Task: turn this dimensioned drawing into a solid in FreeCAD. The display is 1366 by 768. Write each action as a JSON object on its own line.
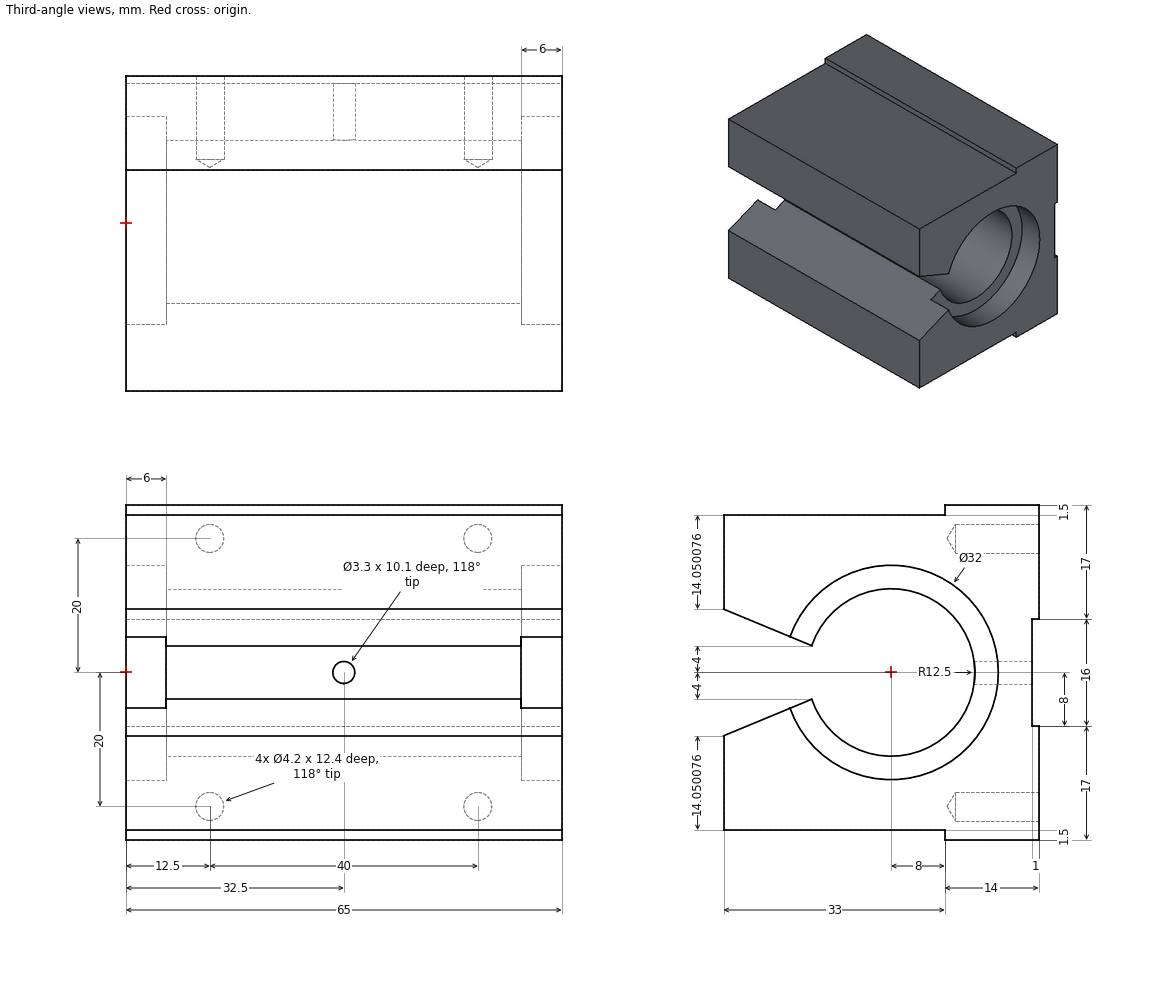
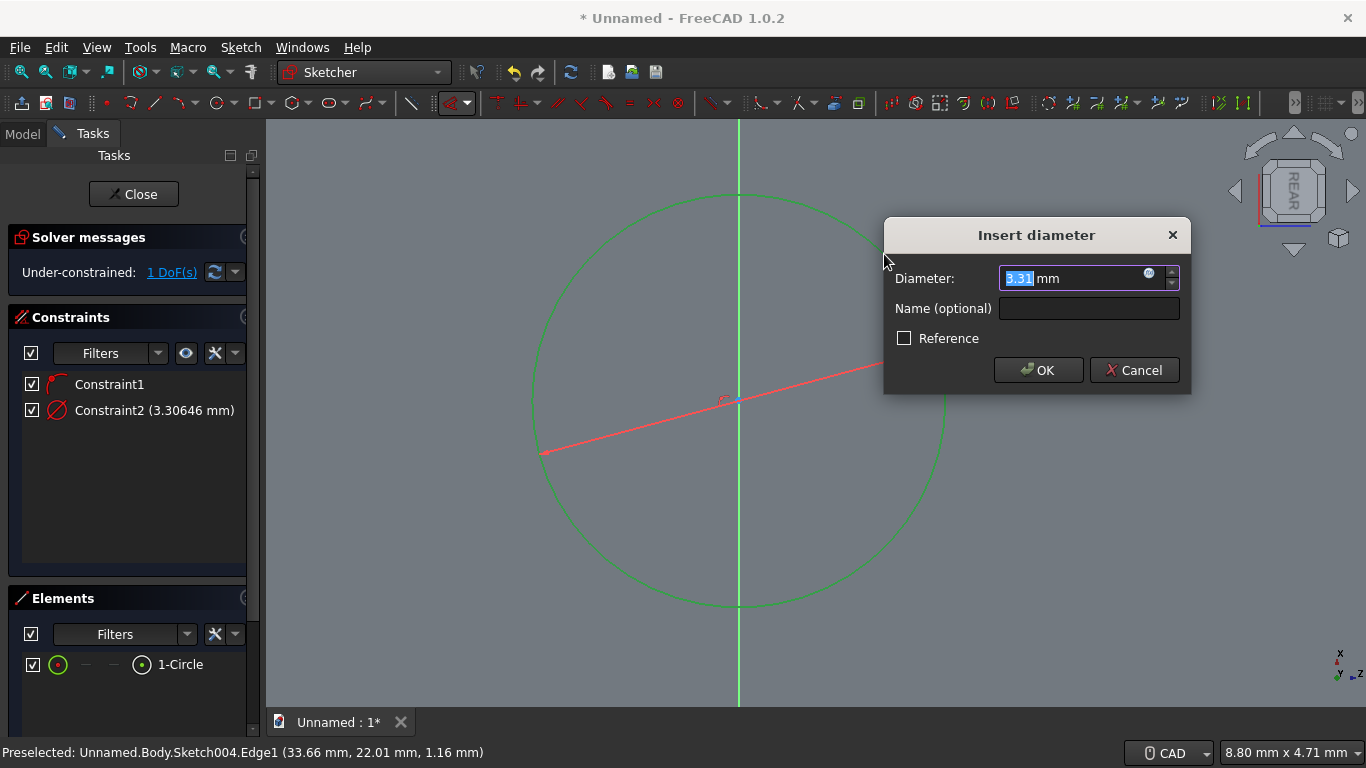
{"action": "type", "text": "3.3"}
{"action": "key", "text": "Return"}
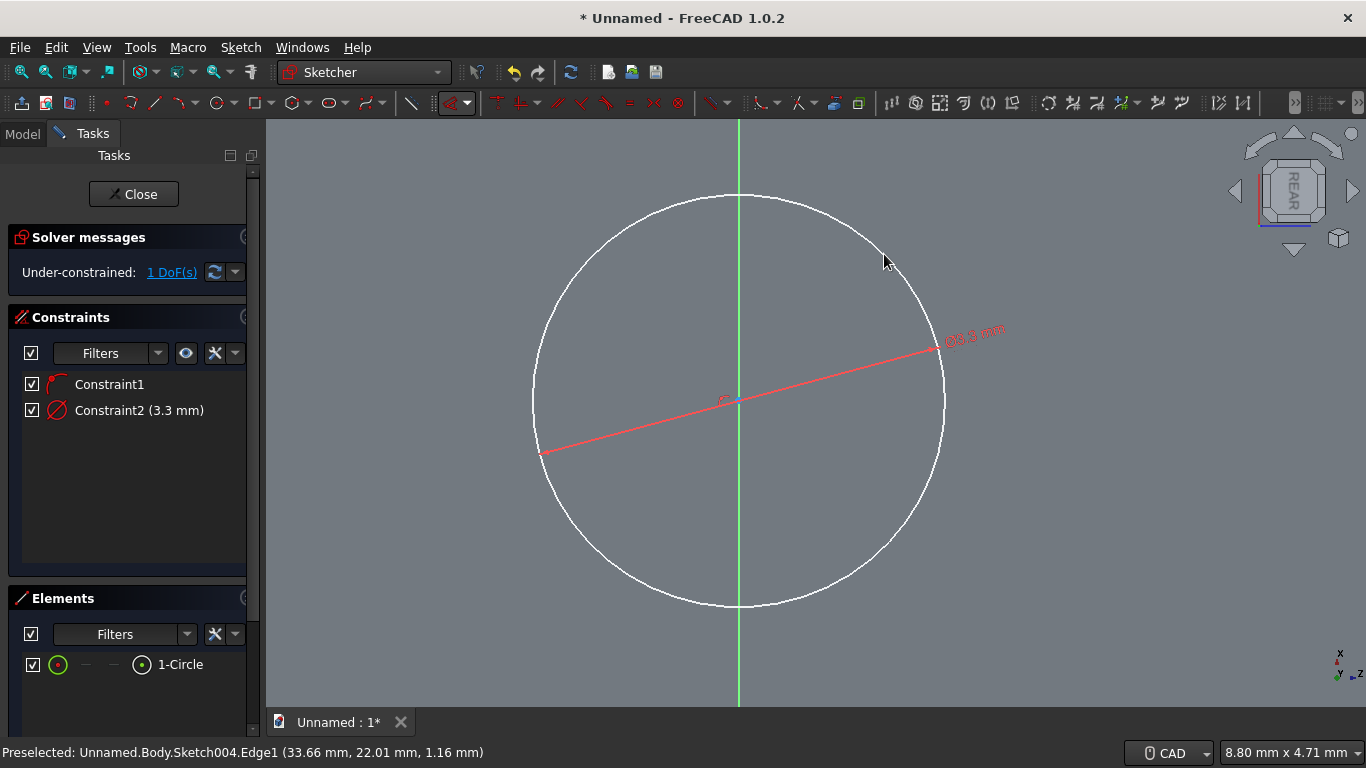
{"action": "left_click", "coordinate": [739, 401]}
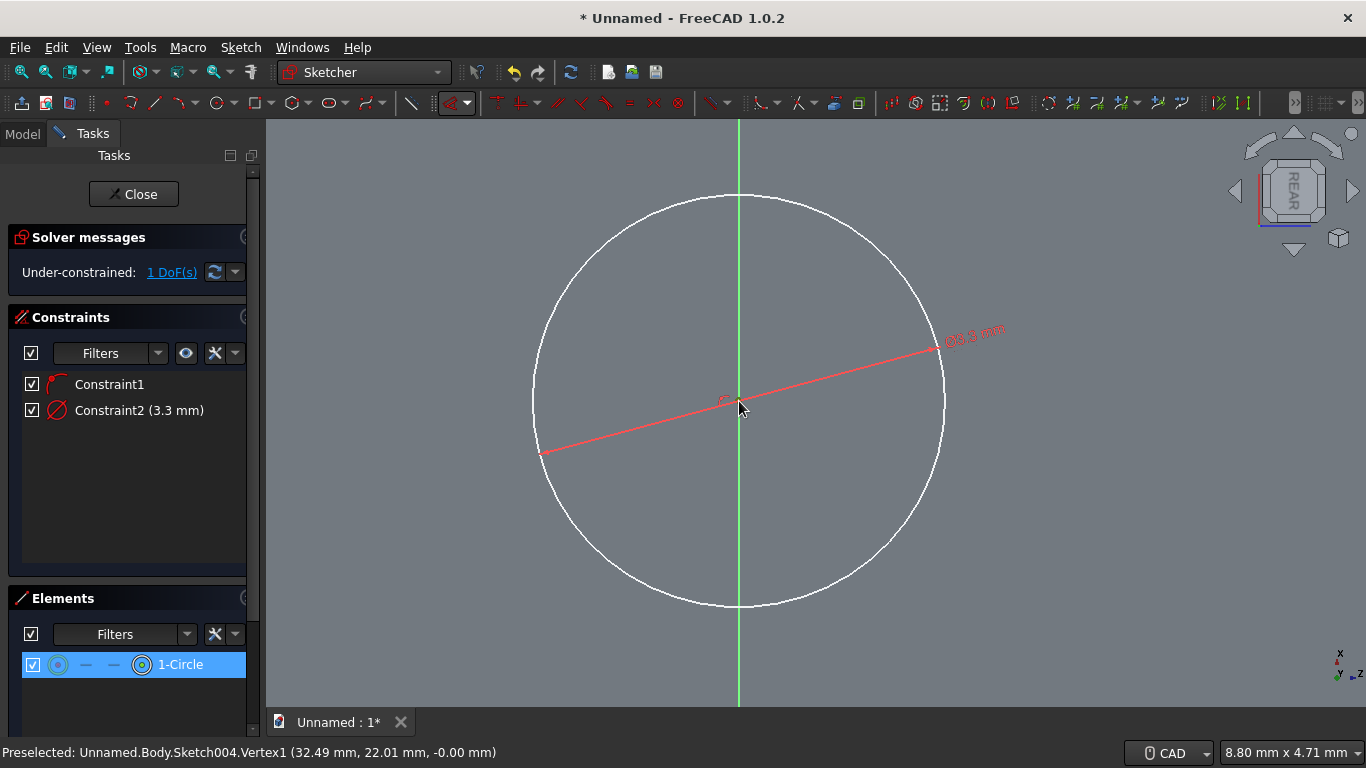
{"action": "key", "text": "i"}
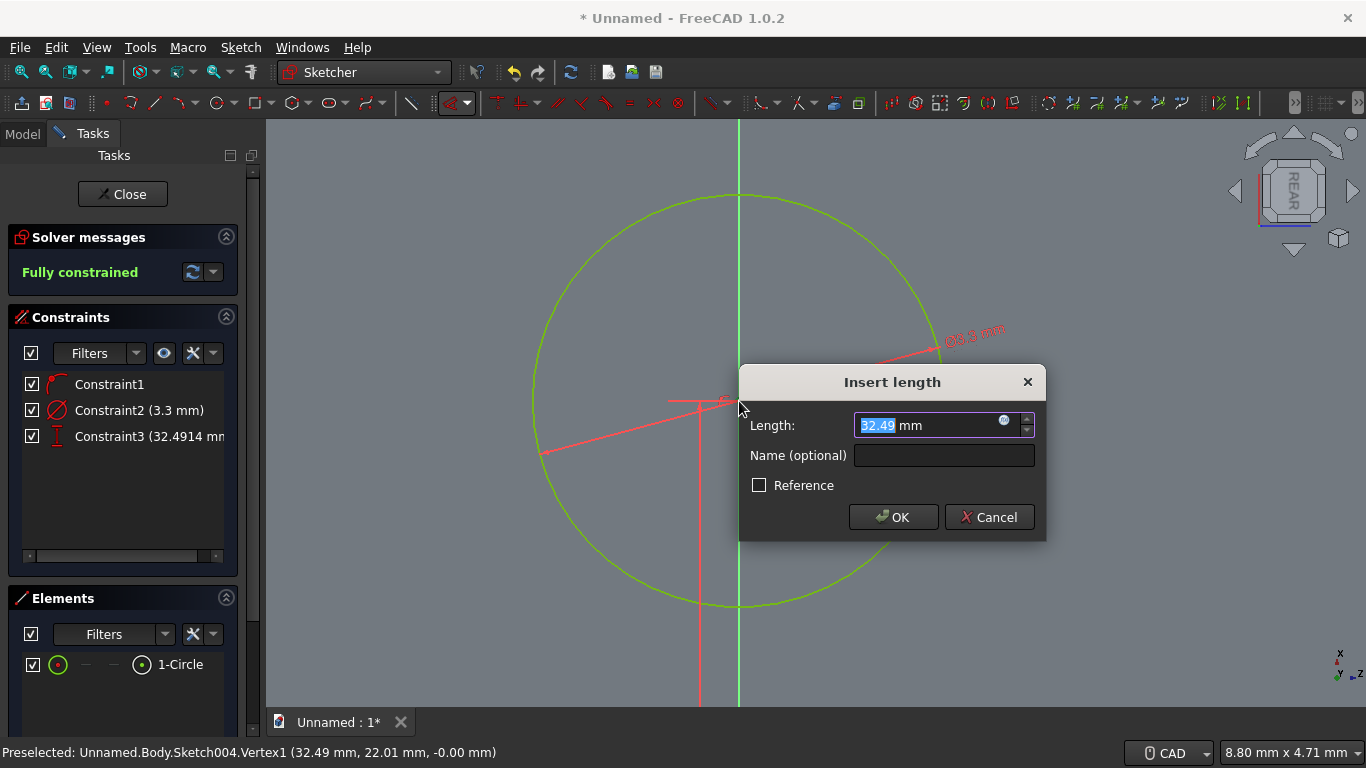
{"action": "type", "text": "32.5"}
{"action": "key", "text": "Return"}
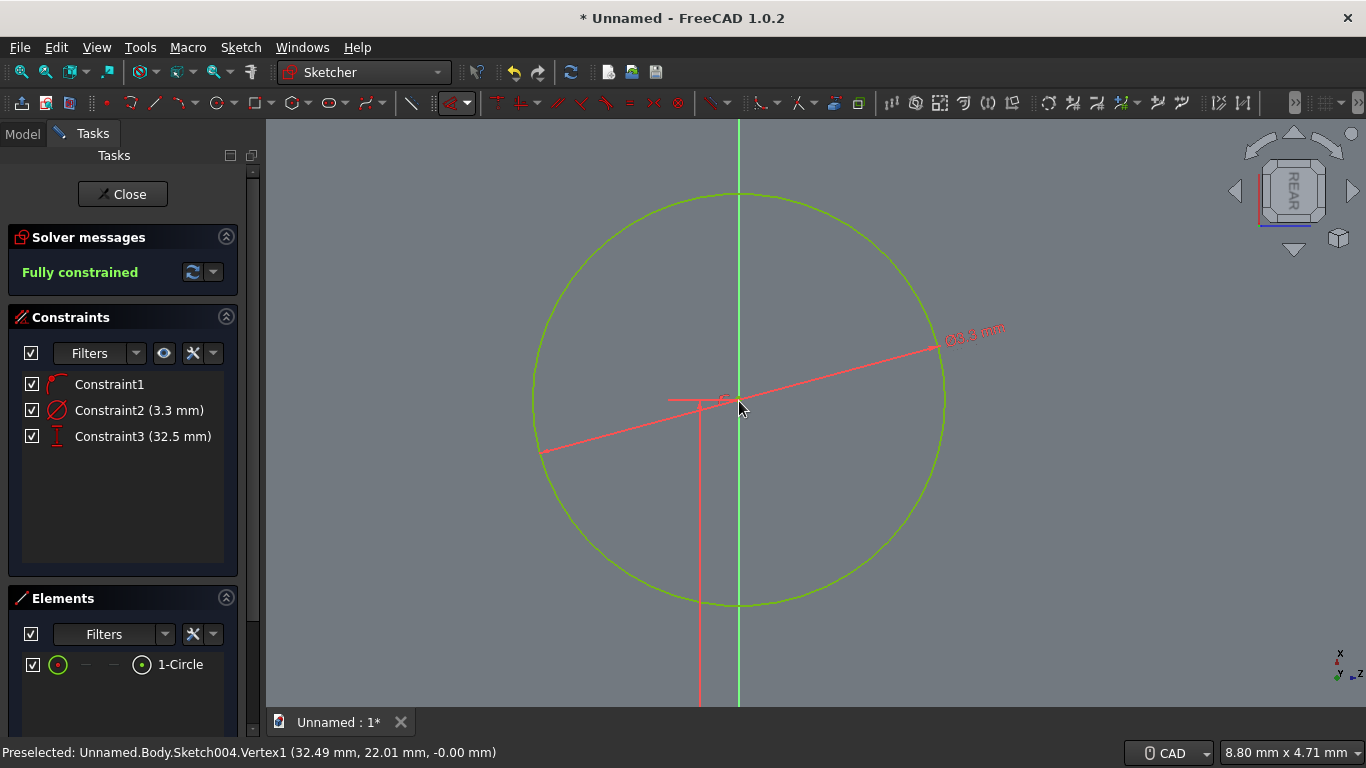
{"action": "left_click", "coordinate": [123, 194]}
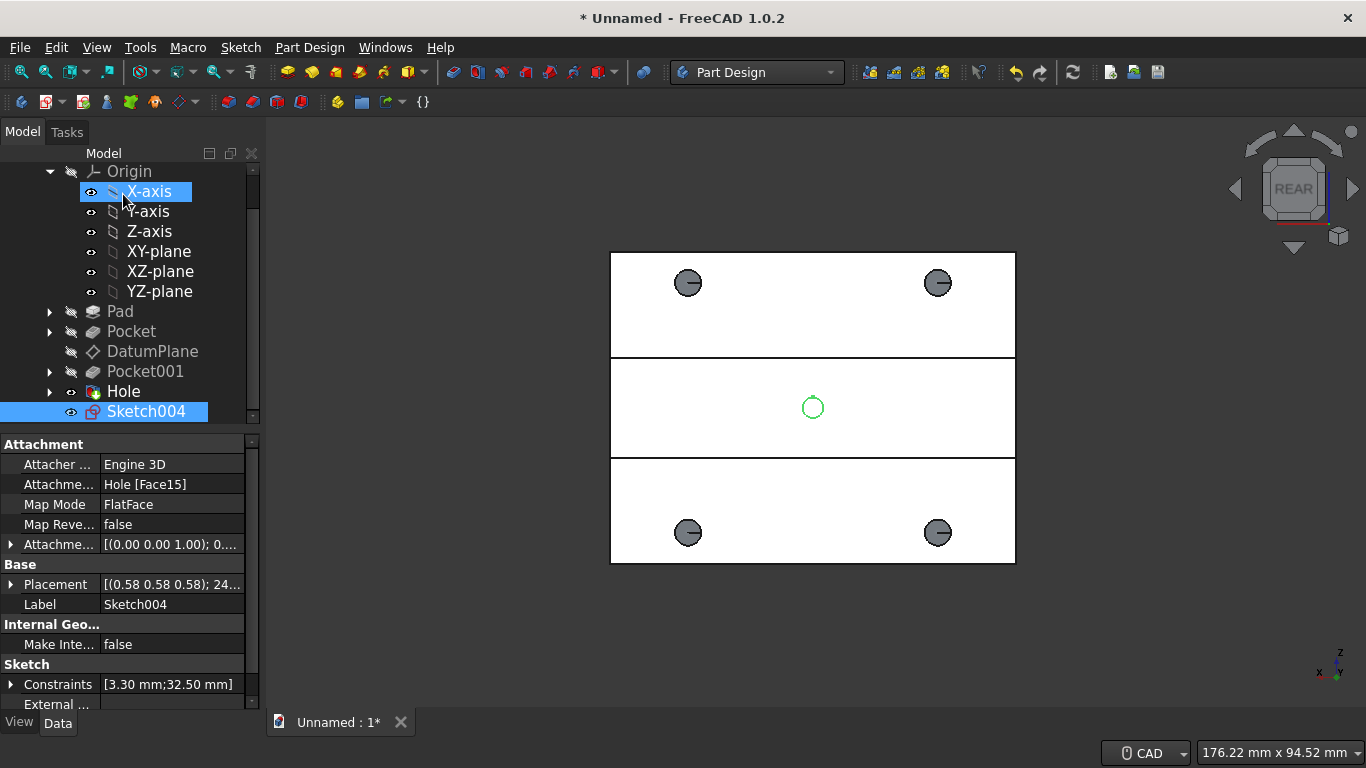
{"action": "left_click", "coordinate": [478, 72]}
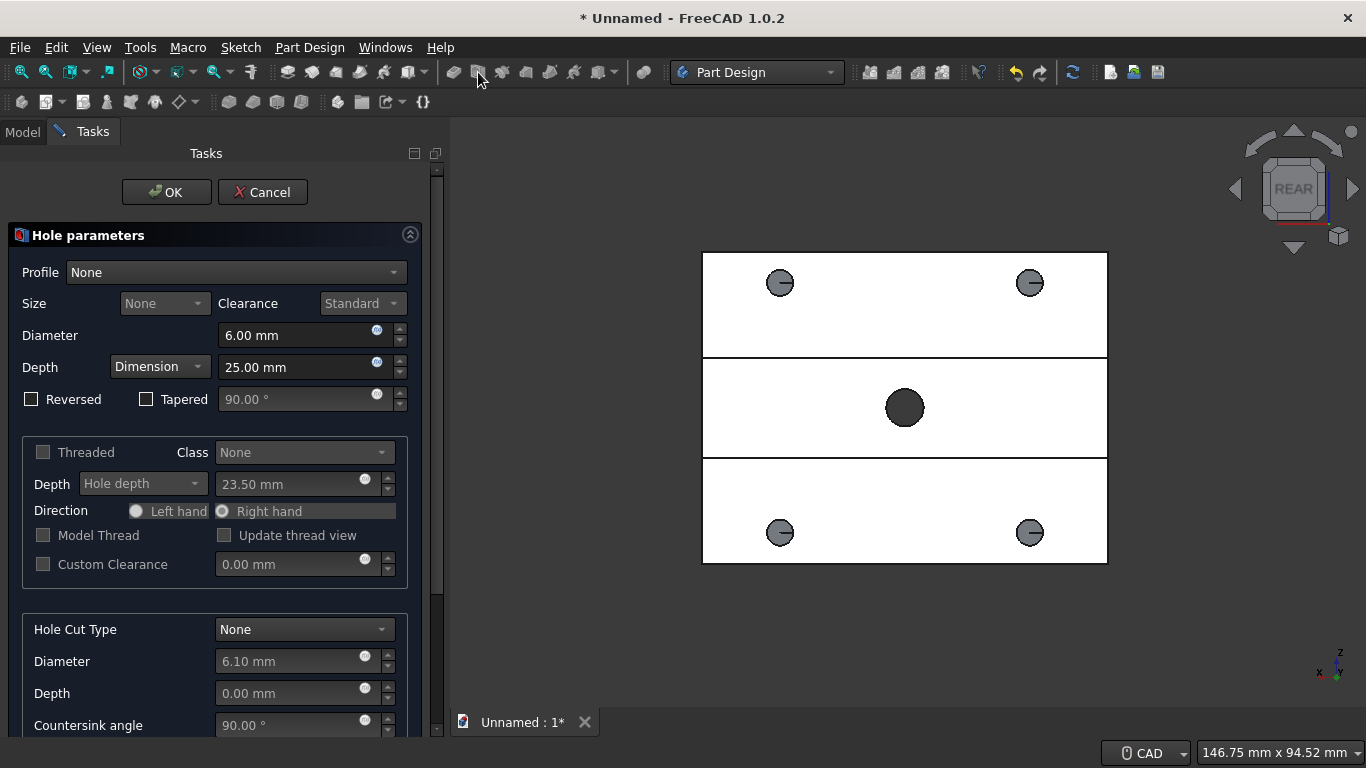
{"action": "triple_click", "coordinate": [305, 335]}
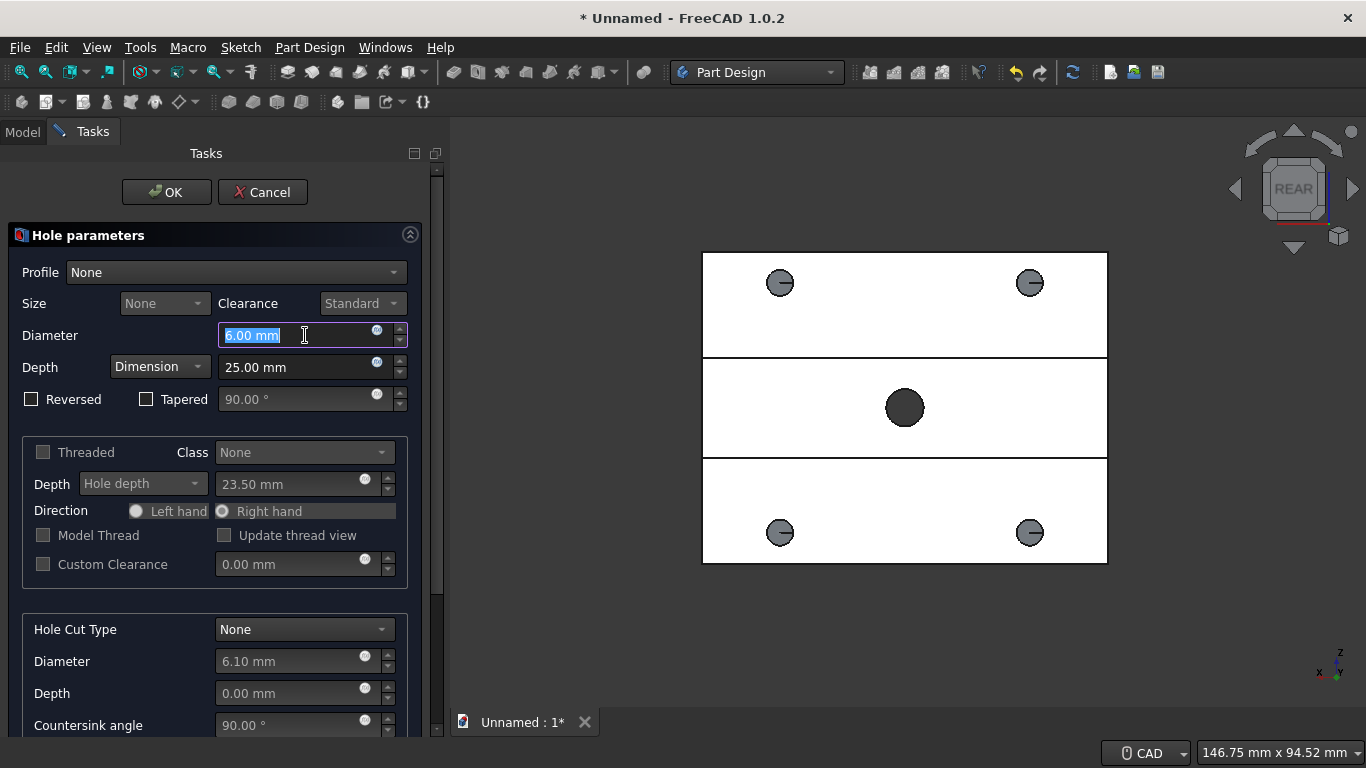
{"action": "type", "text": "3.3"}
{"action": "key", "text": "Tab"}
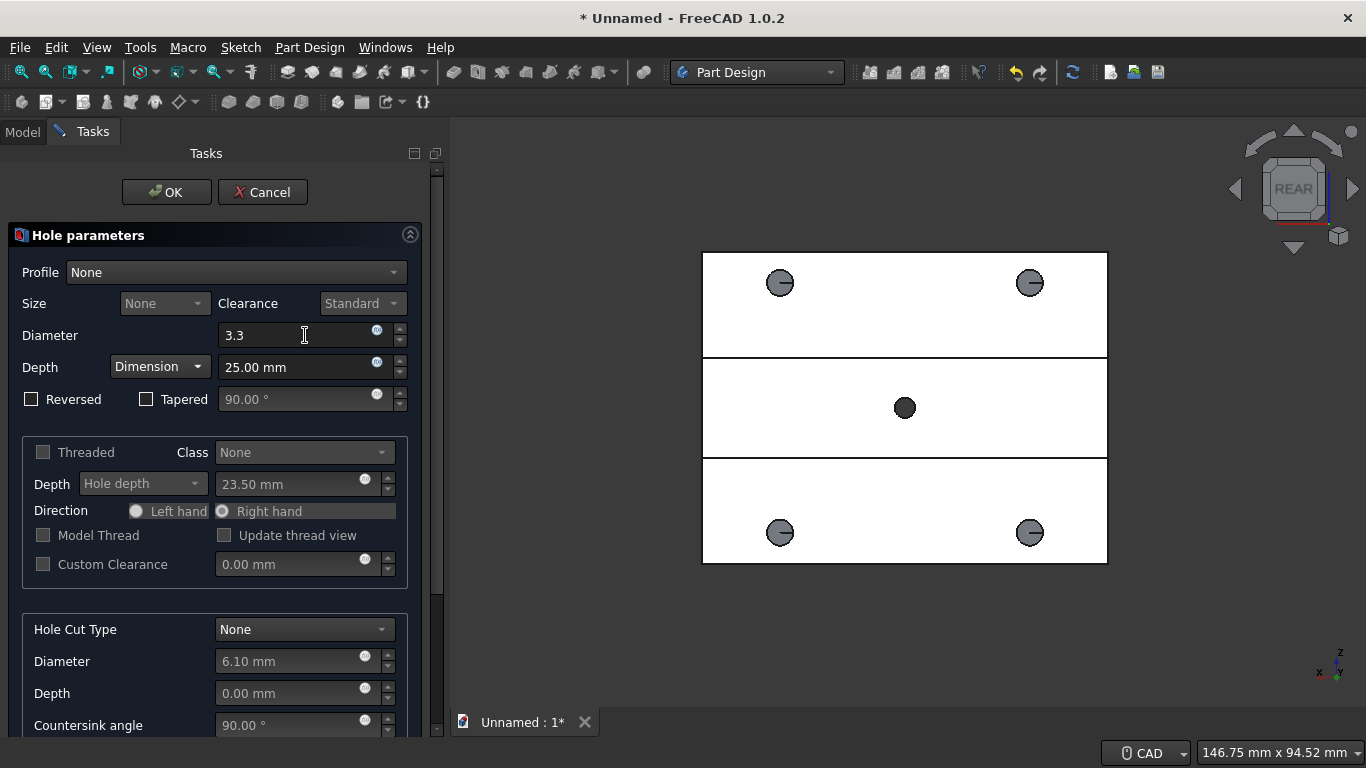
{"action": "triple_click", "coordinate": [305, 367]}